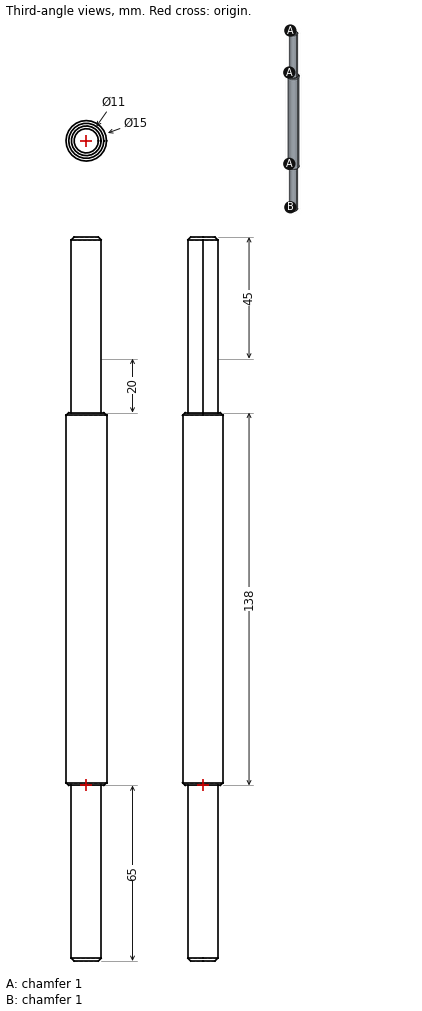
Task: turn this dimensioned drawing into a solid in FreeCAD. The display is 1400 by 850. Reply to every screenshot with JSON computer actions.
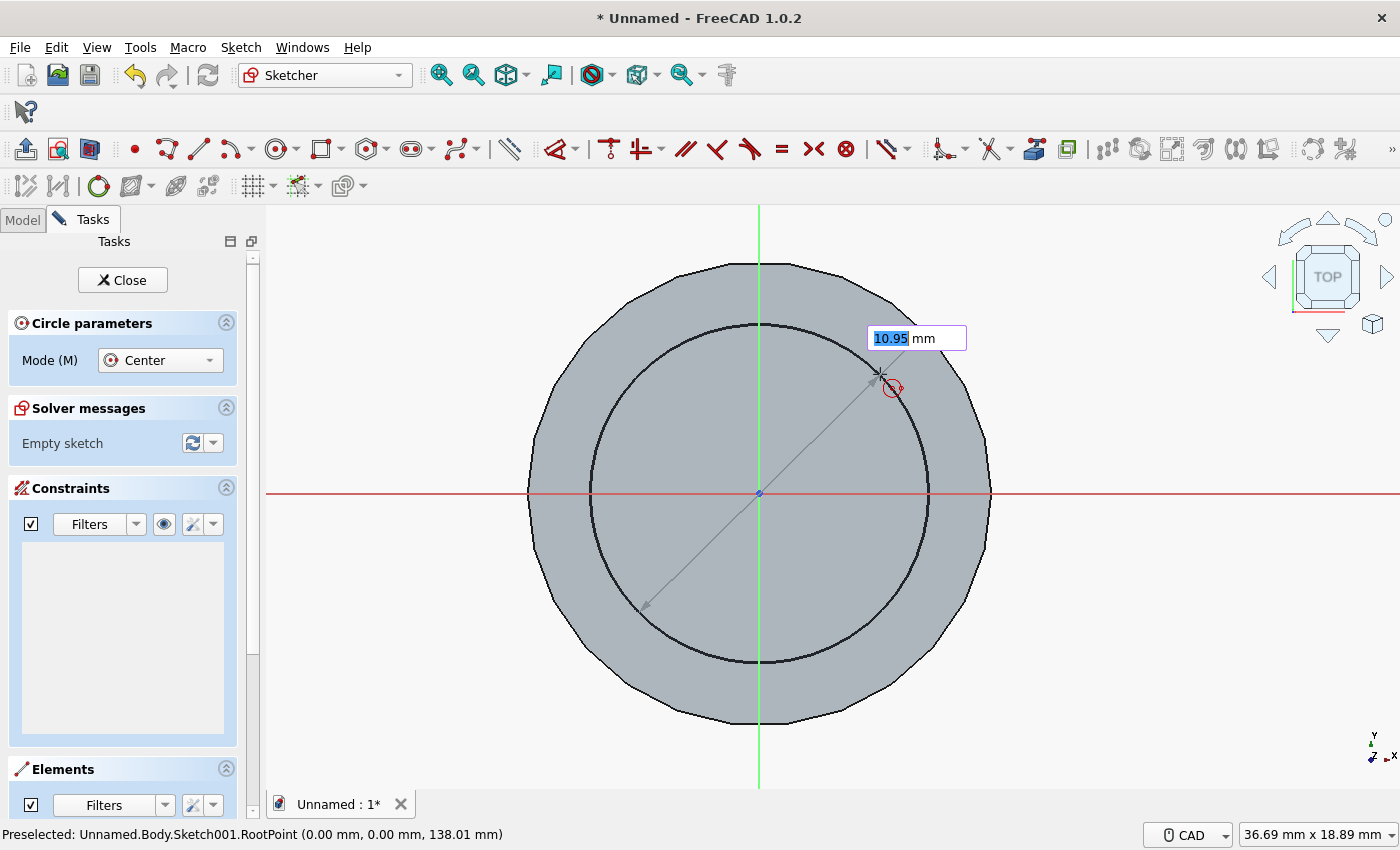
{"action": "type", "text": "11"}
{"action": "key", "text": "Return"}
{"action": "key", "text": "Escape"}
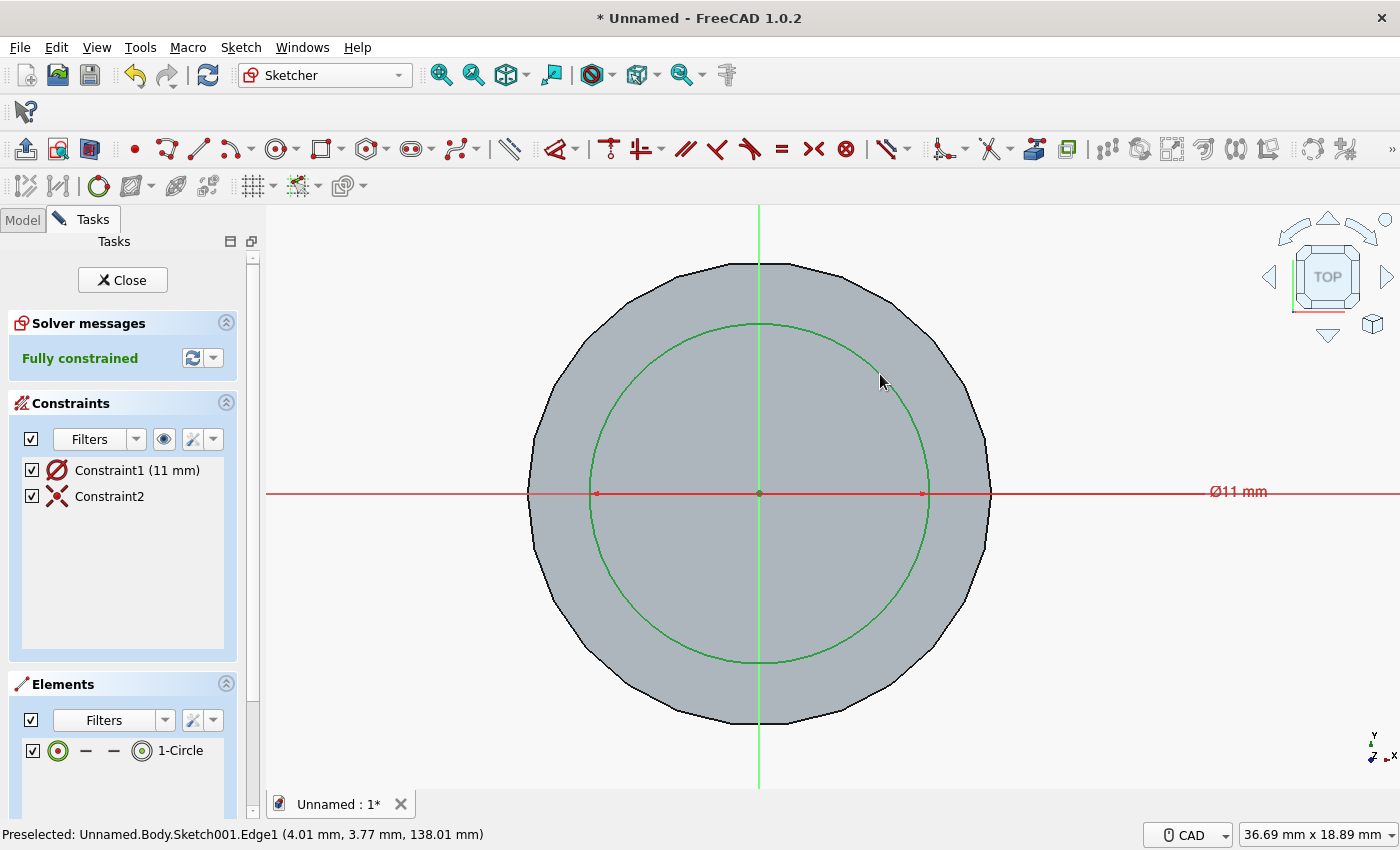
{"action": "left_click", "coordinate": [123, 280]}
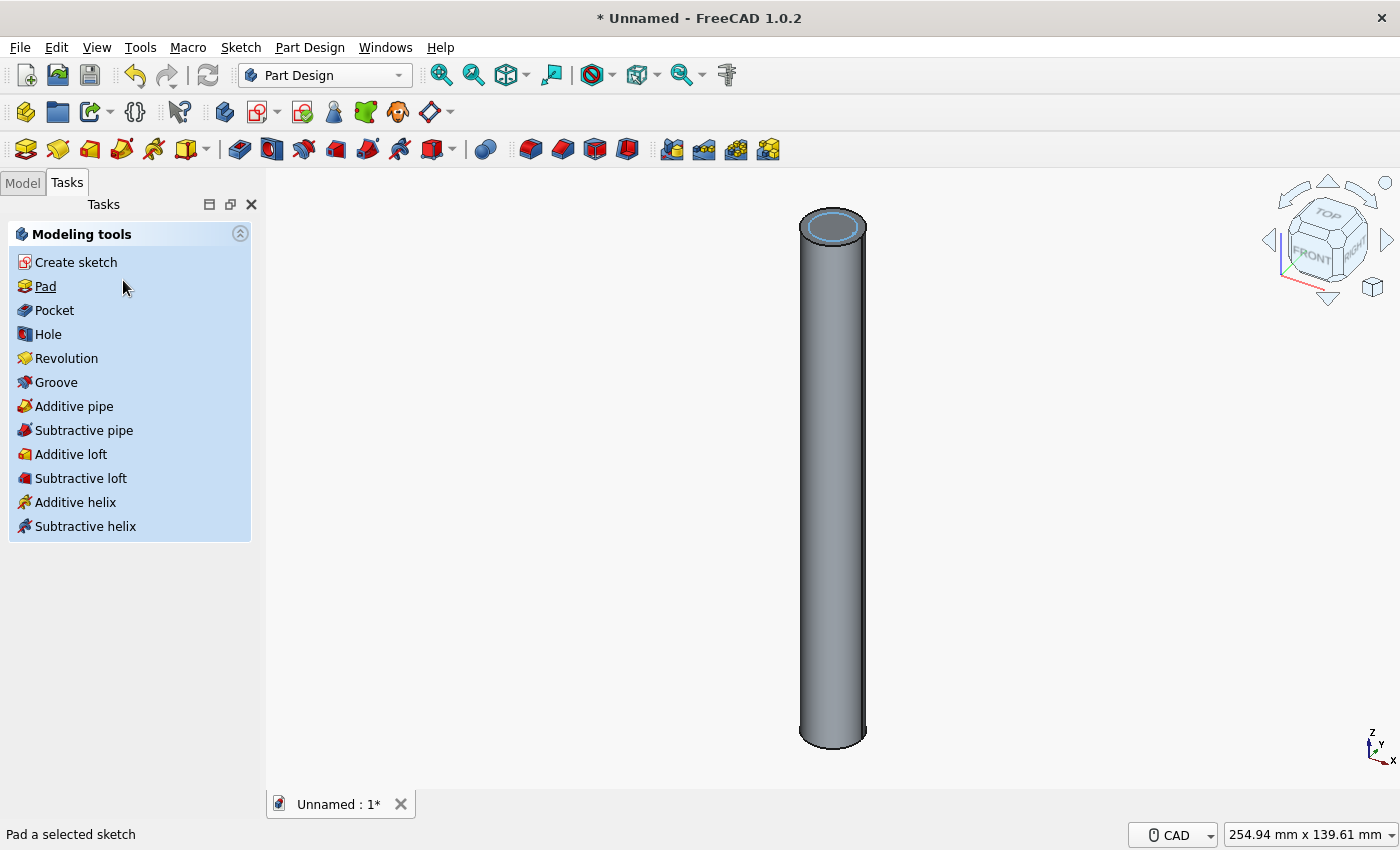
{"action": "left_click", "coordinate": [26, 150]}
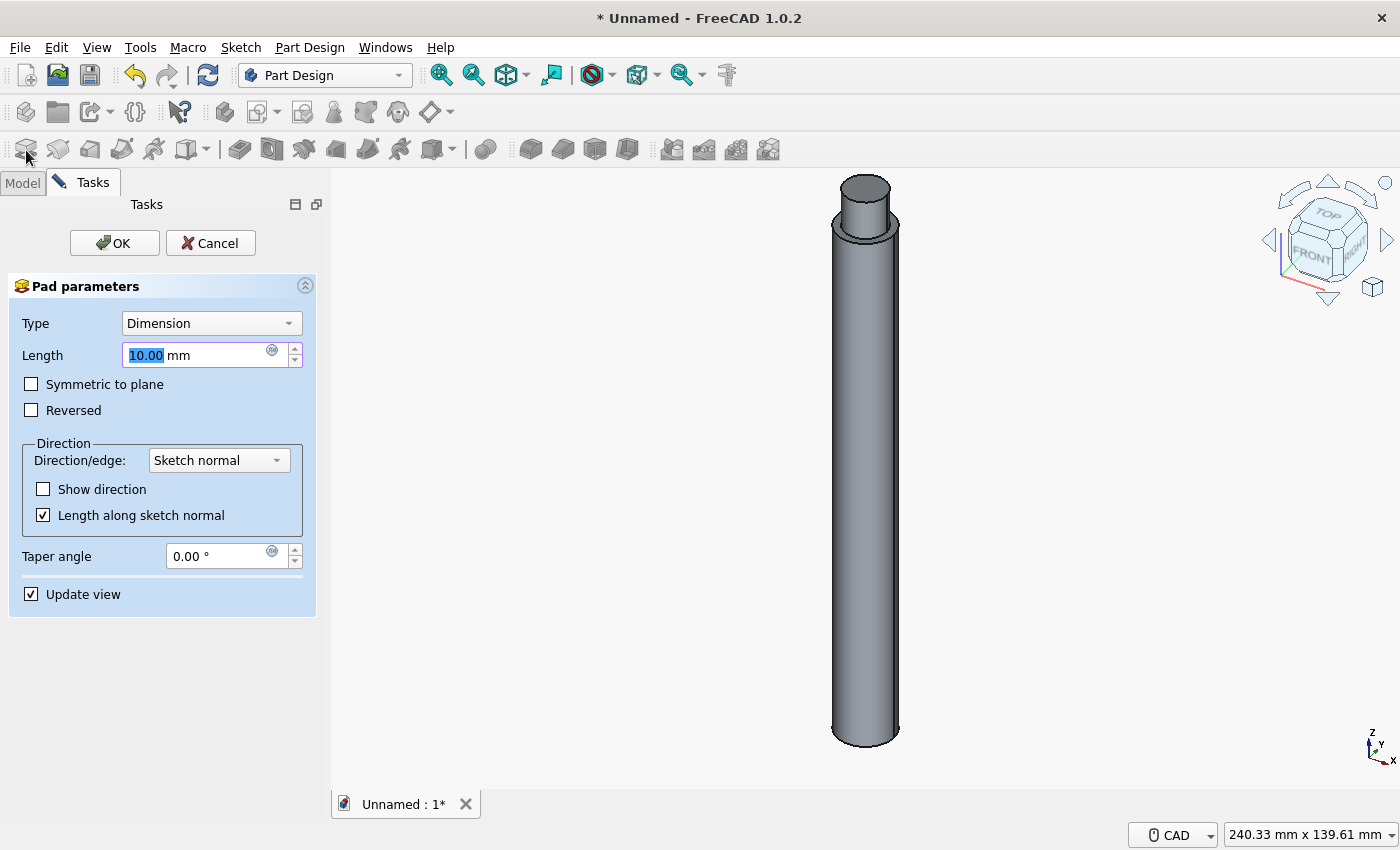
{"action": "type", "text": "20"}
{"action": "key", "text": "Tab"}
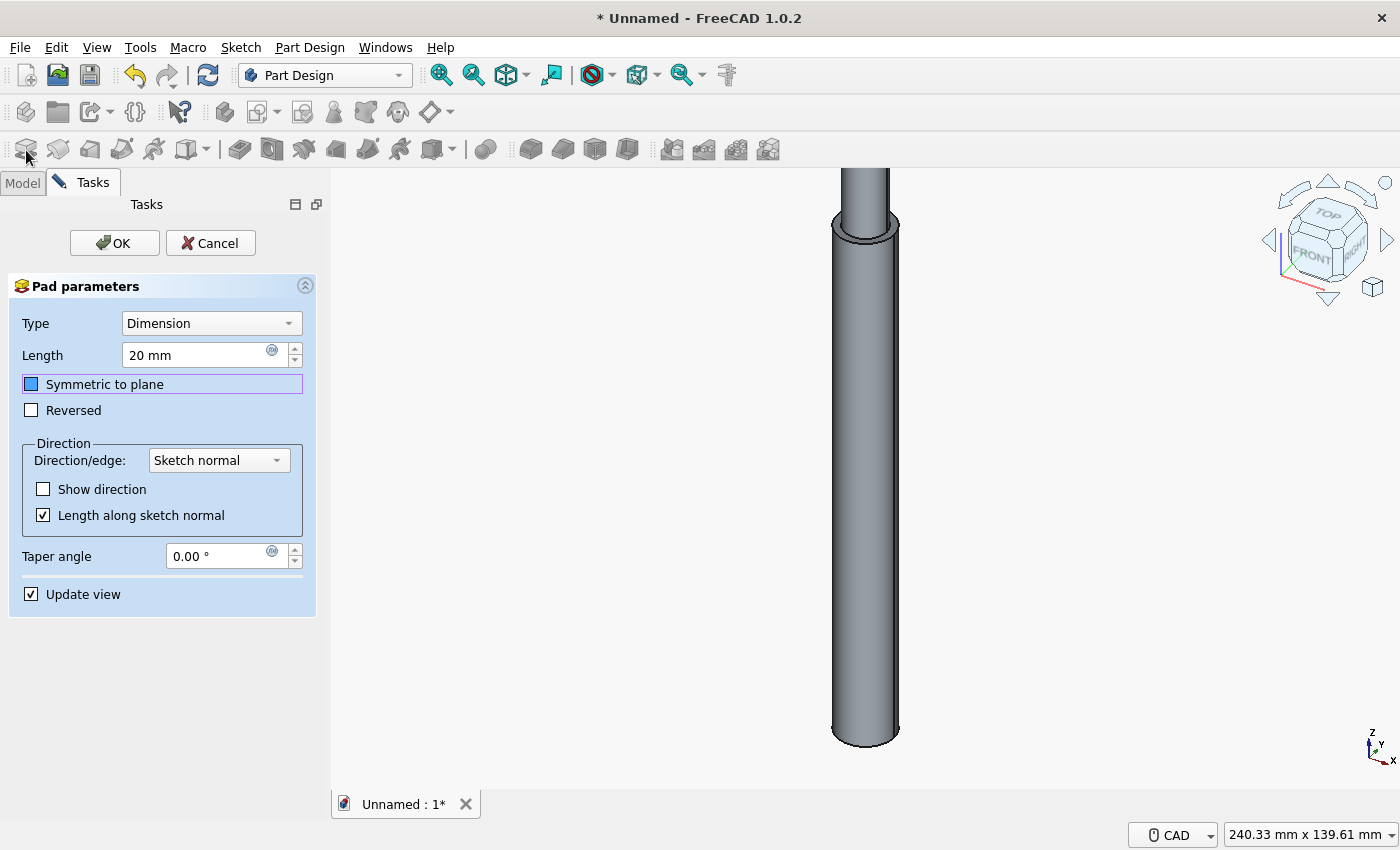
{"action": "left_click", "coordinate": [115, 243]}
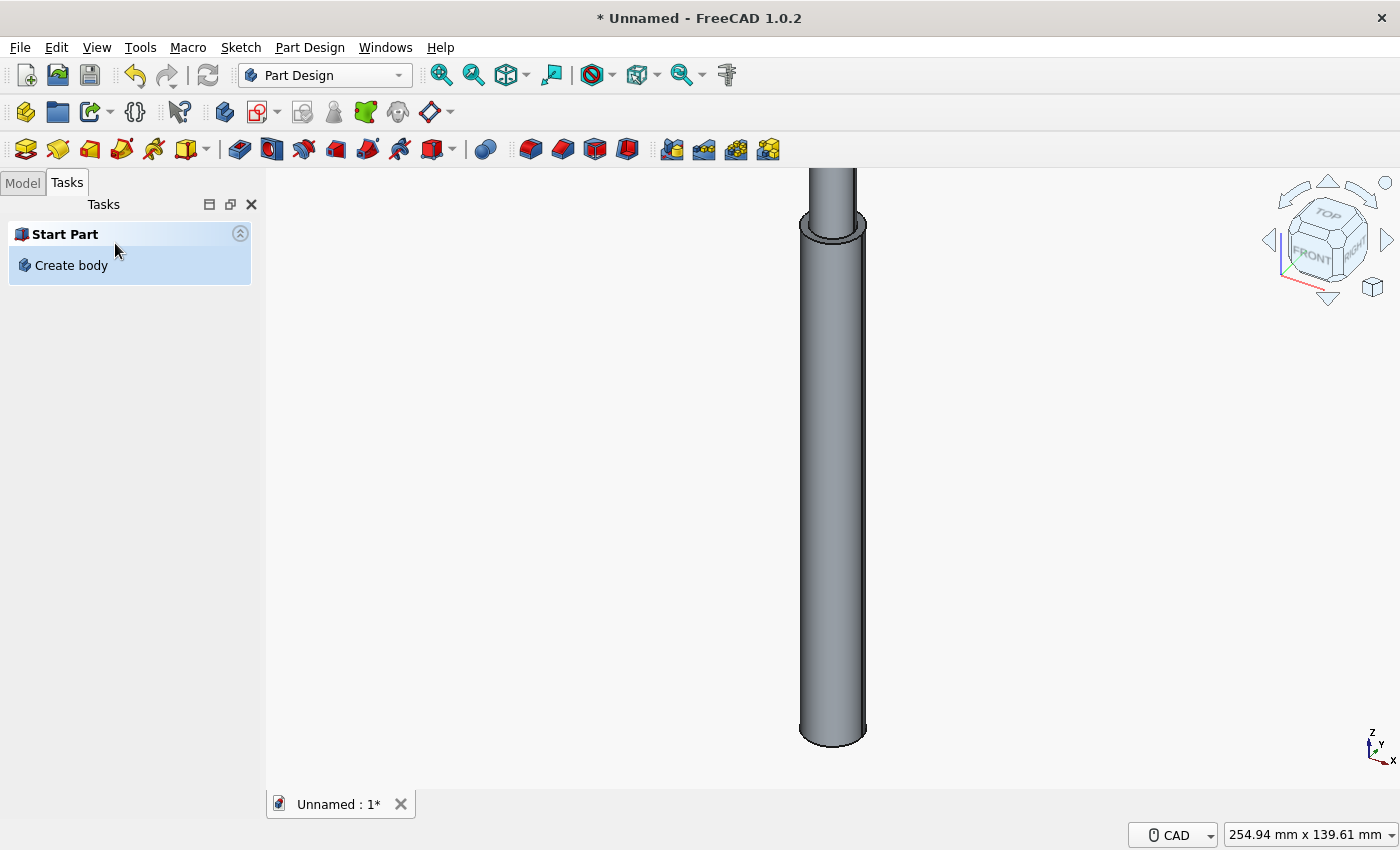
{"action": "key", "text": "v f"}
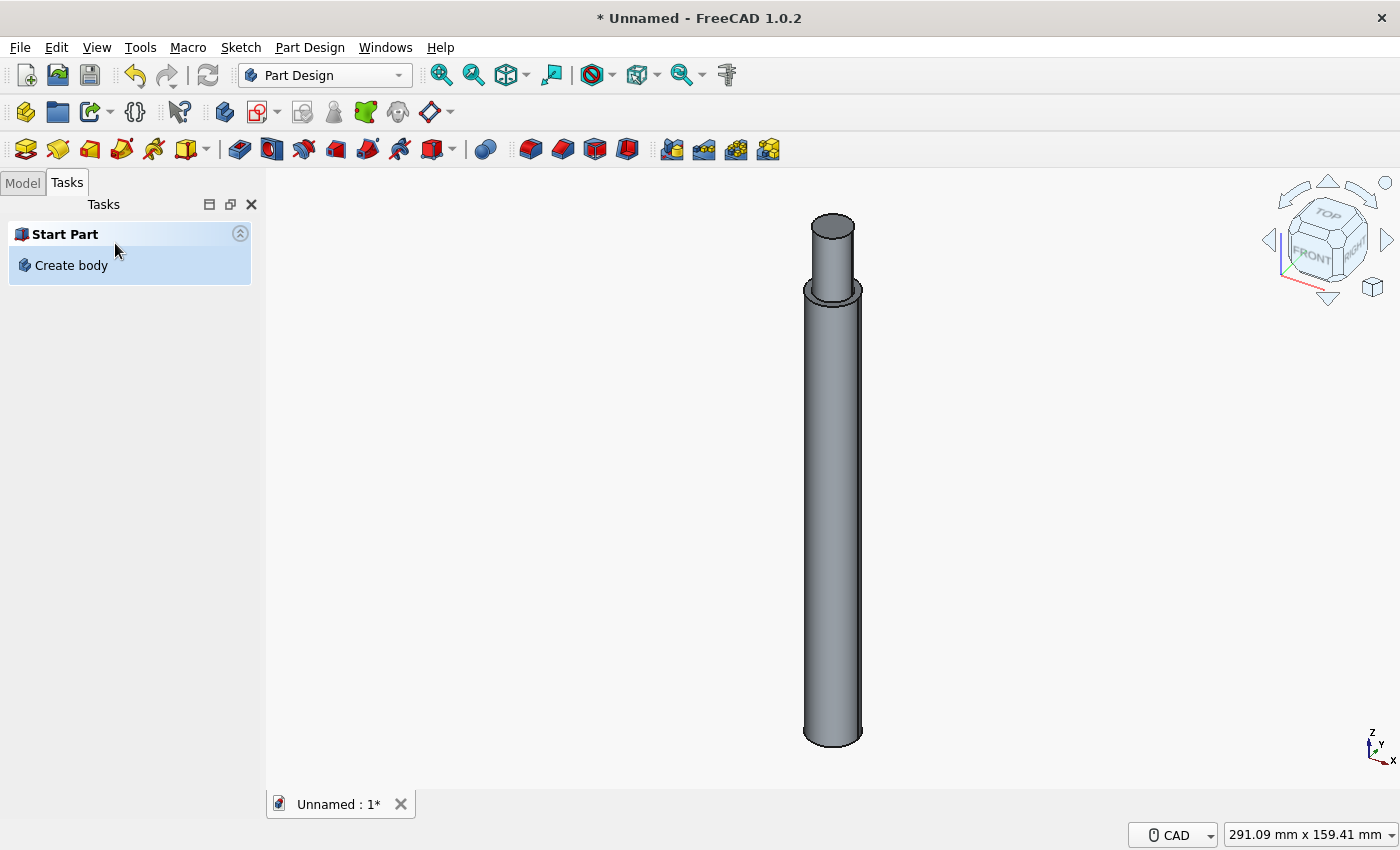
{"action": "left_click", "coordinate": [833, 225]}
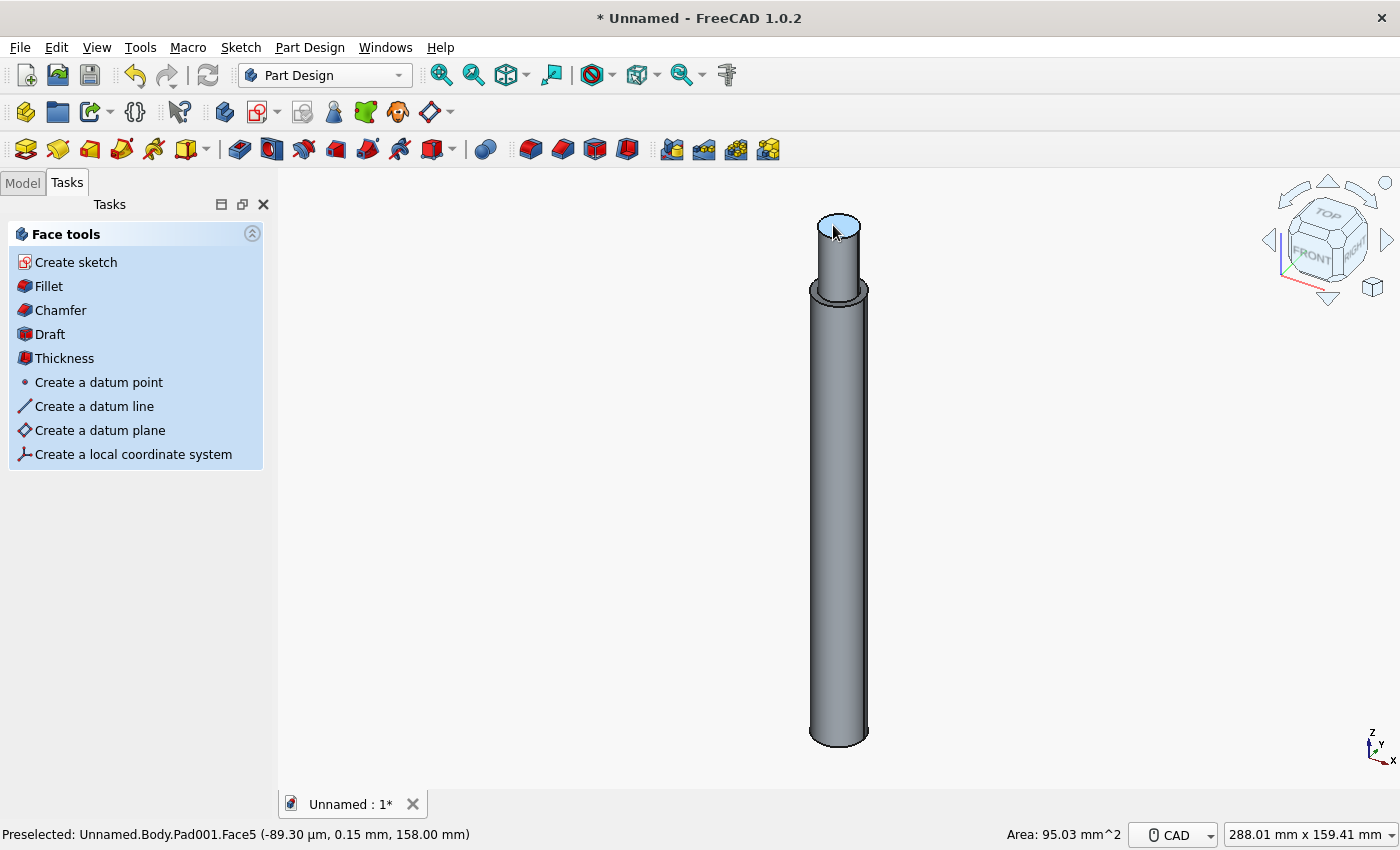
{"action": "left_click", "coordinate": [258, 112]}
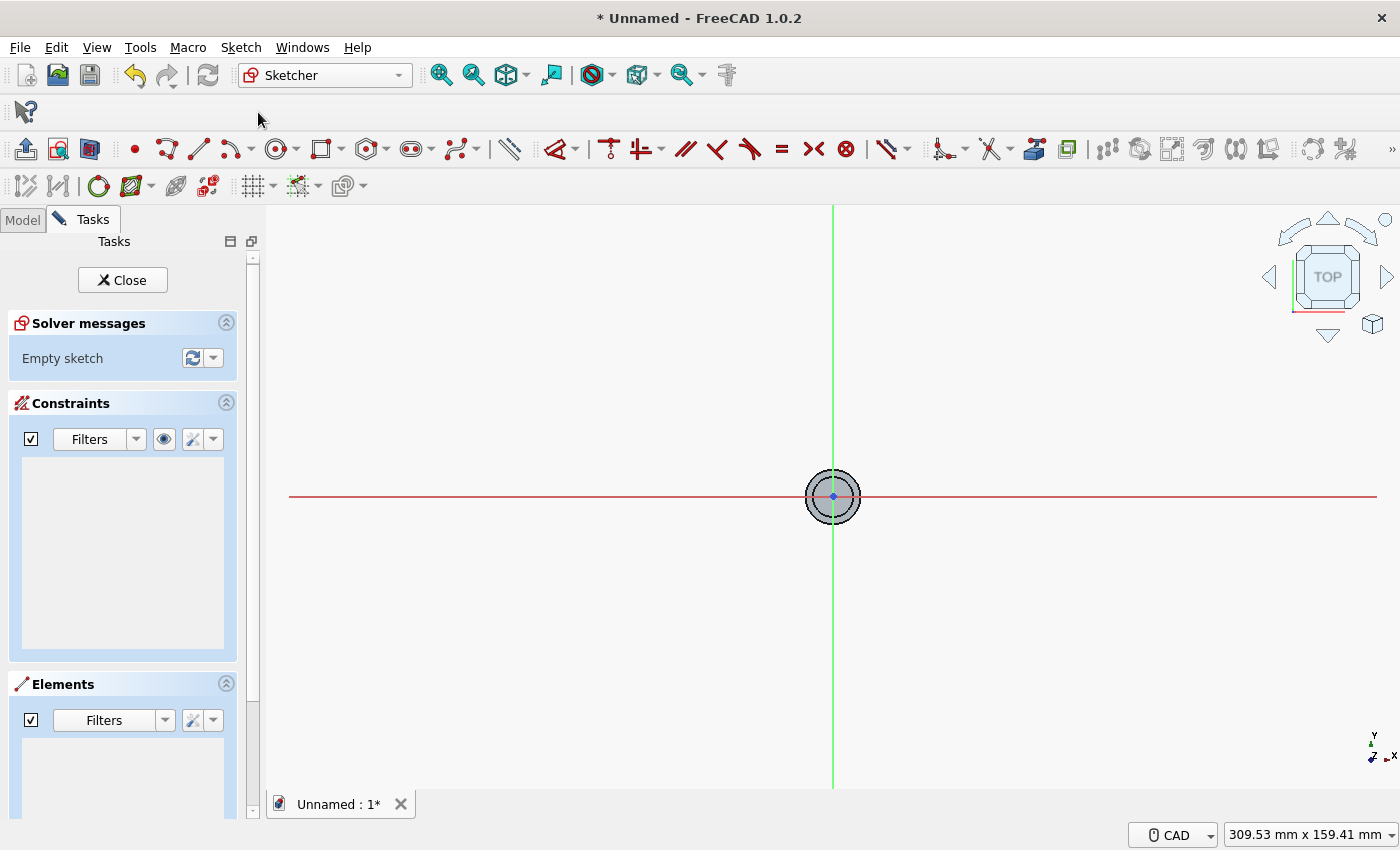
{"action": "scroll", "coordinate": [842, 497], "scroll_direction": "up", "scroll_amount": 11}